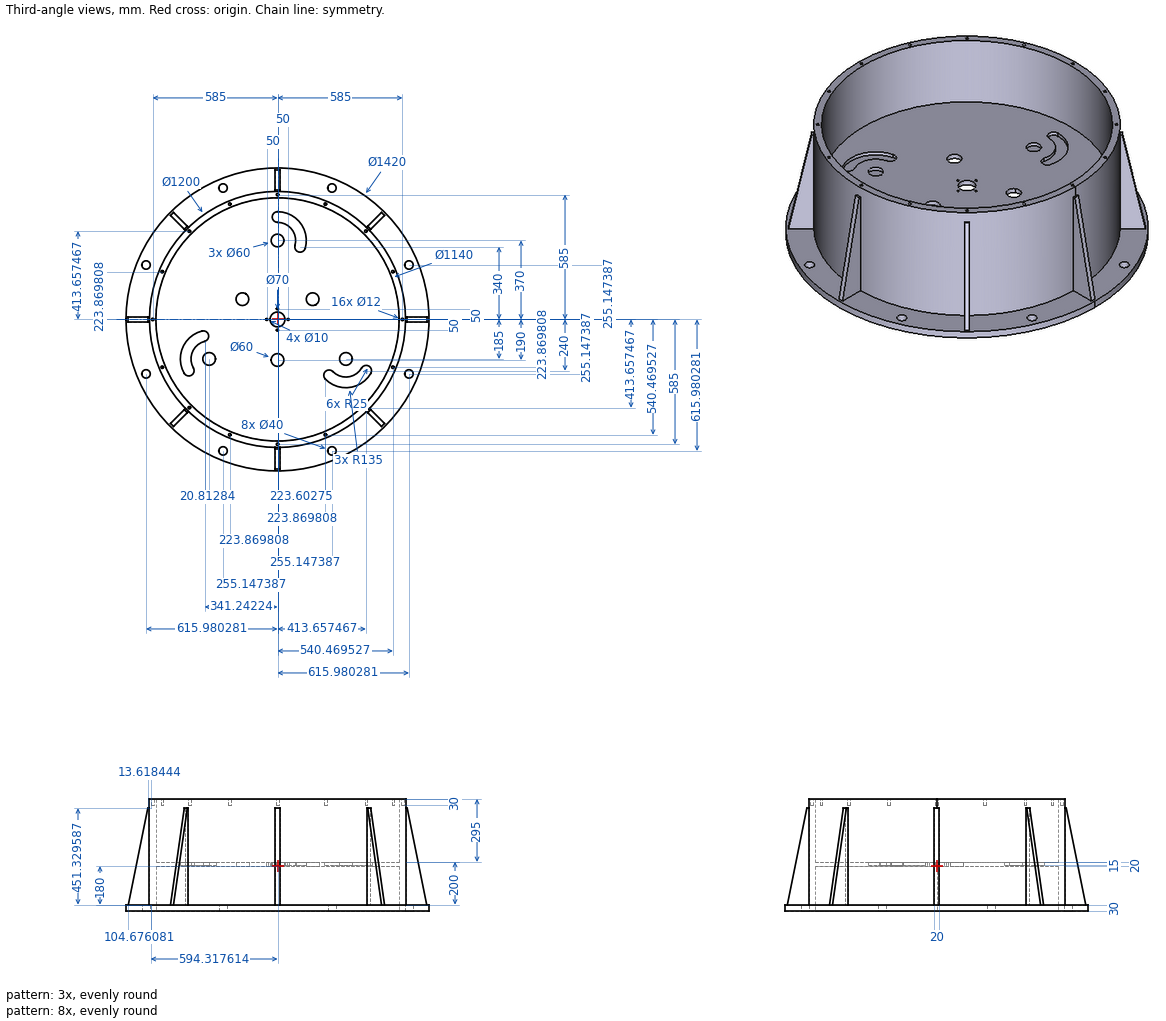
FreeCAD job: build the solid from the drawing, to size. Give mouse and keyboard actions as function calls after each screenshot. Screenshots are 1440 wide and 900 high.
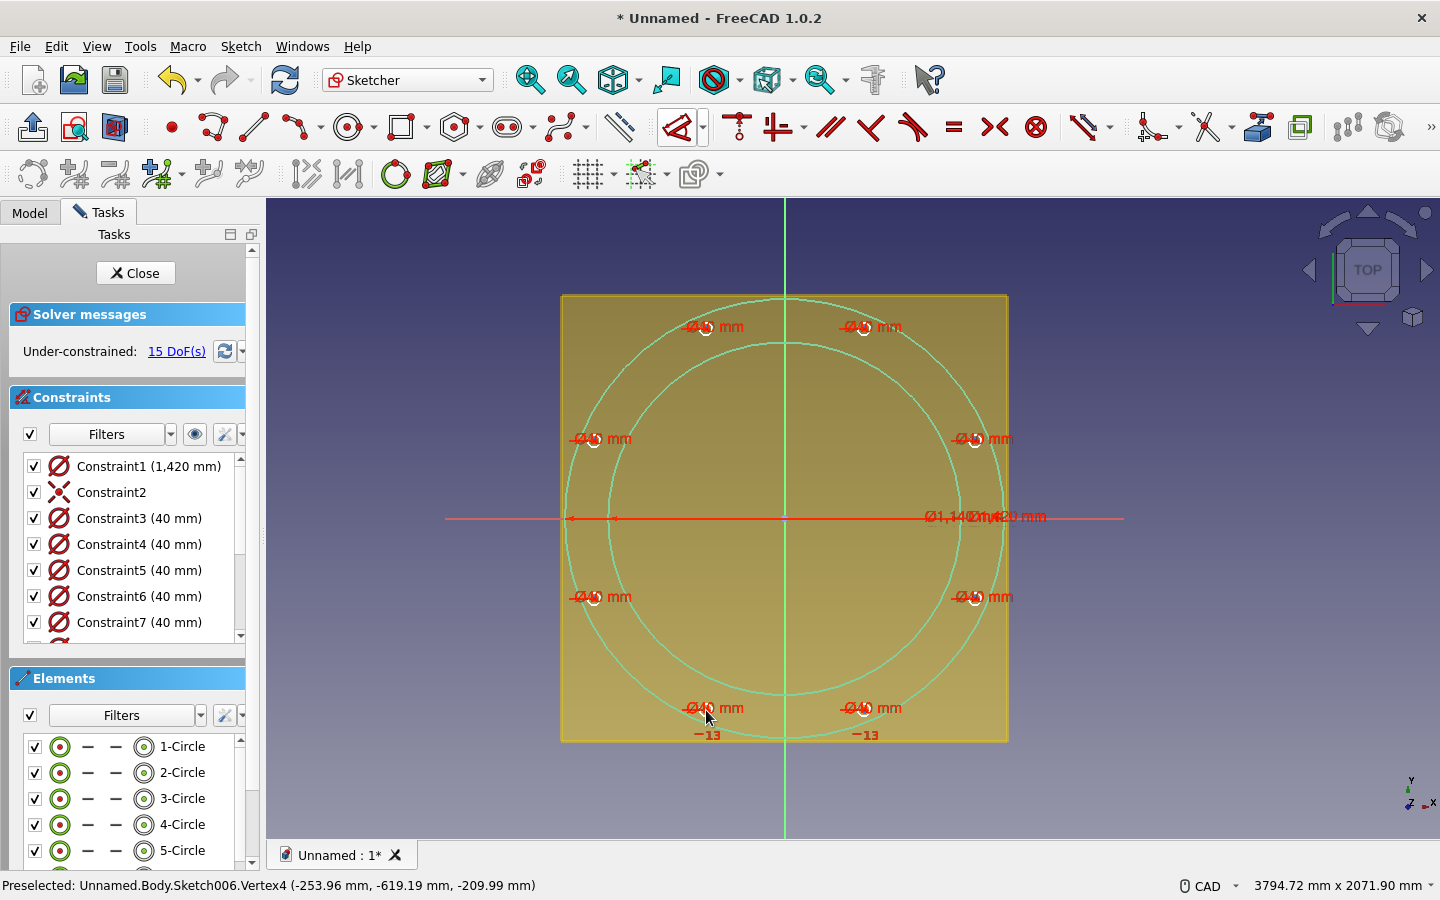
click(975, 599)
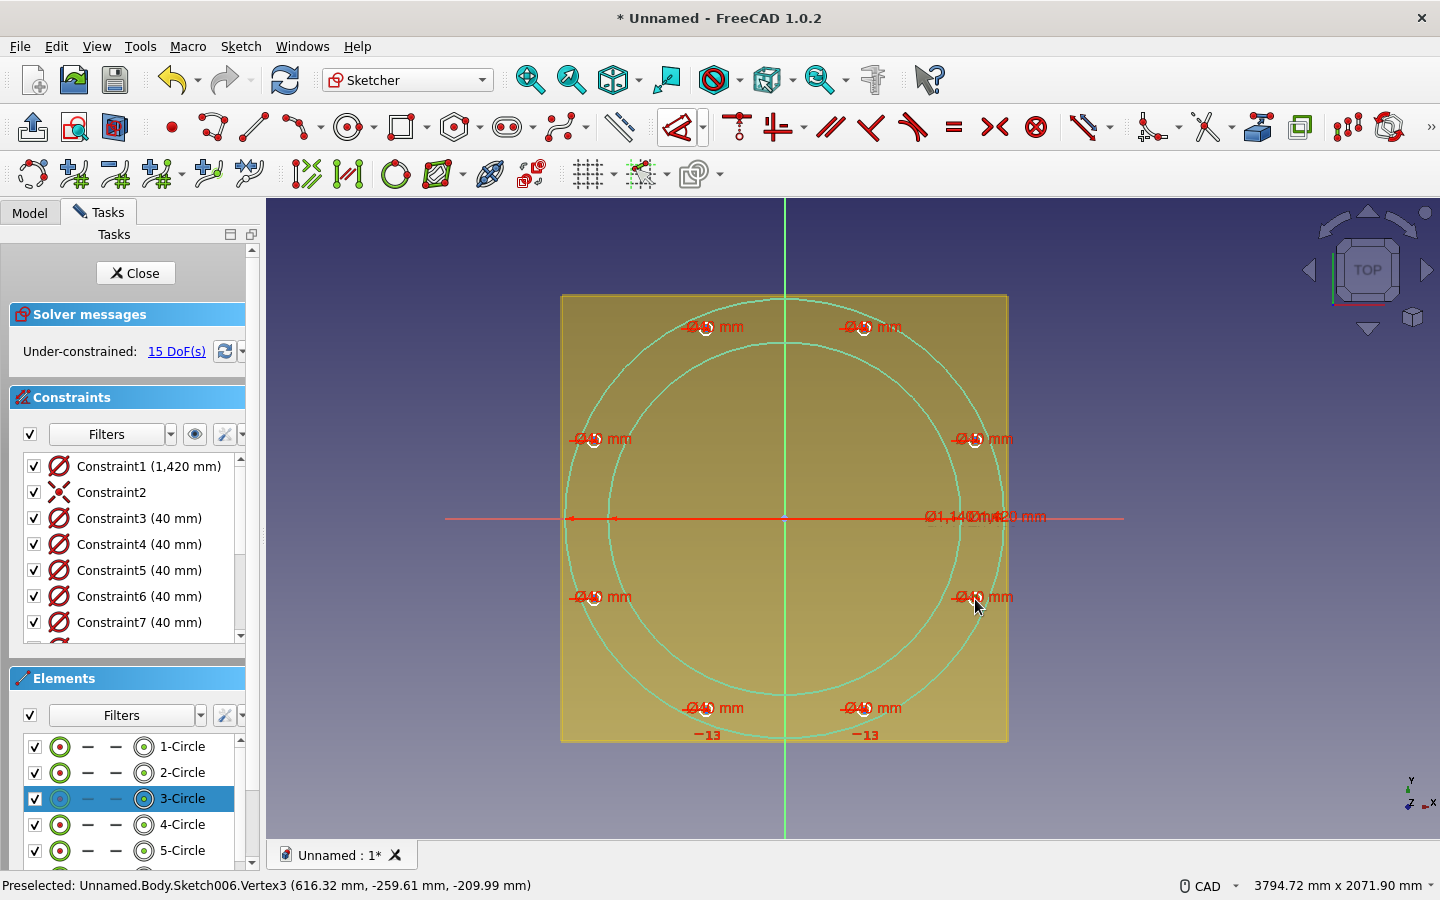
click(594, 599)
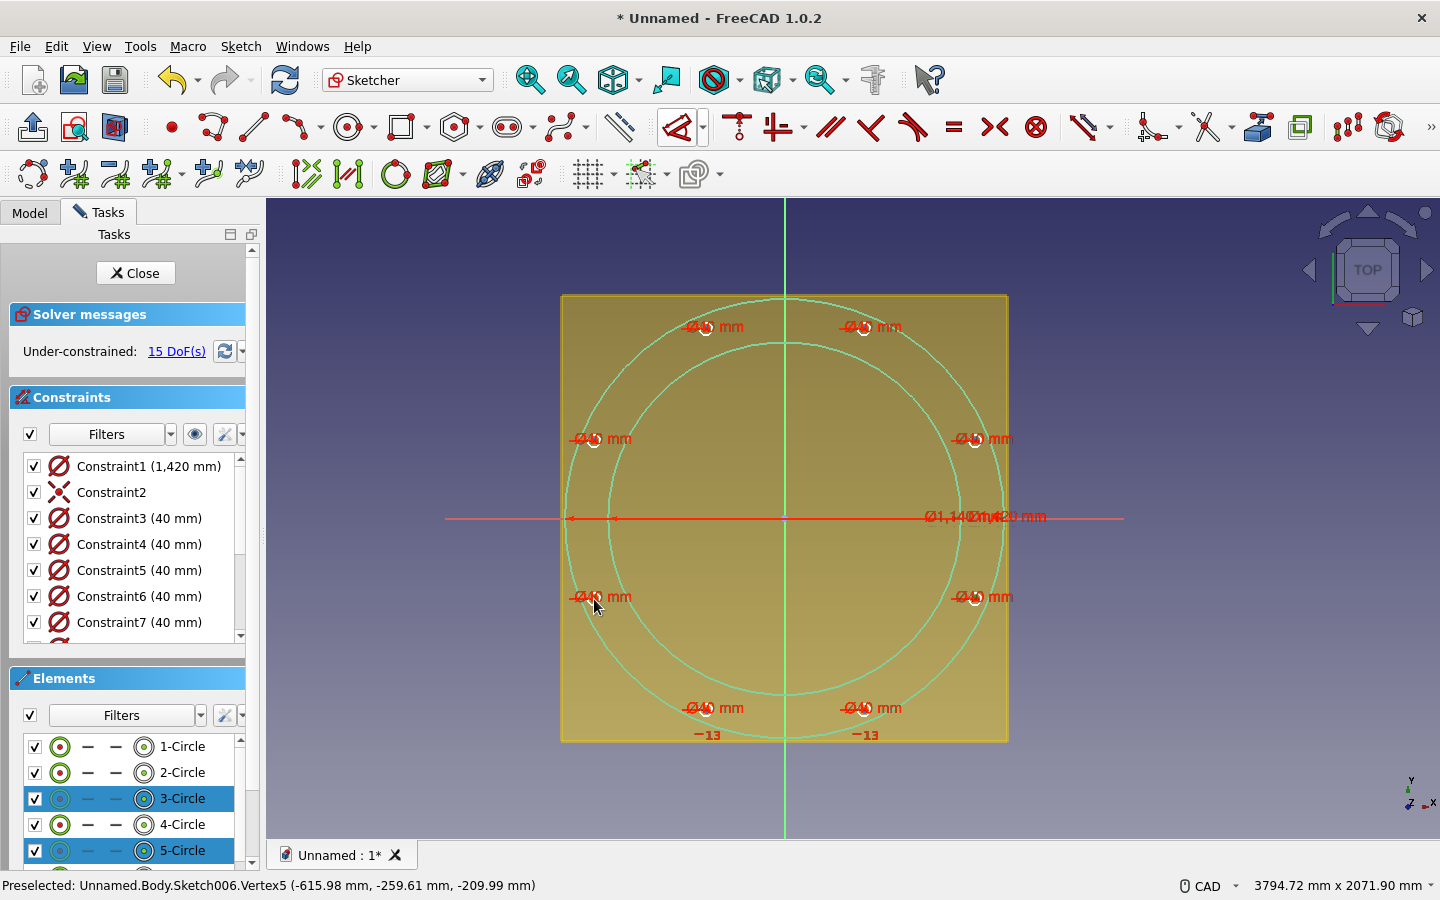
key(h)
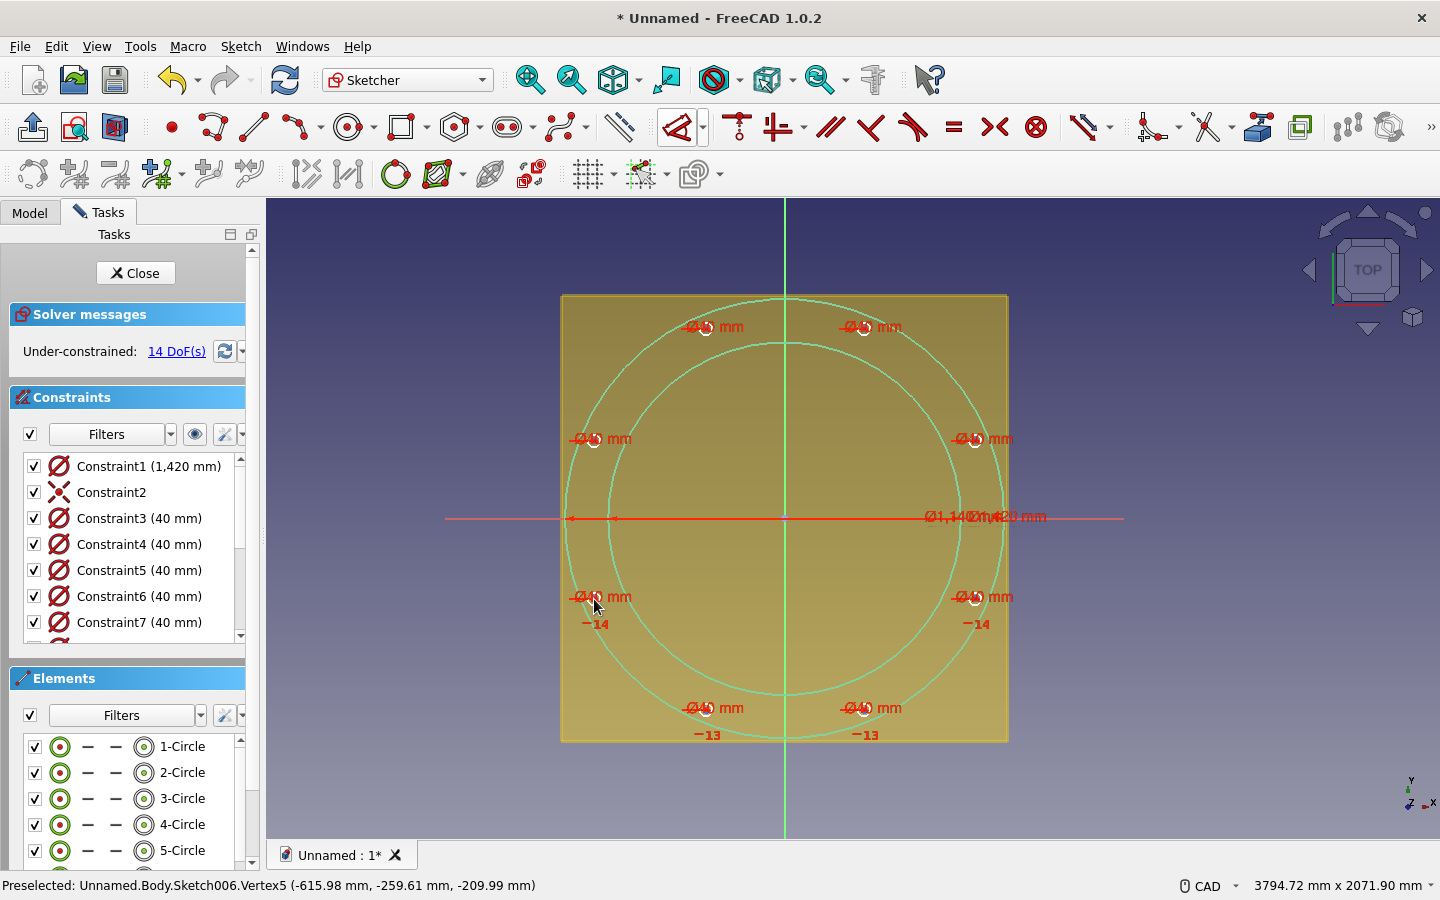
click(975, 599)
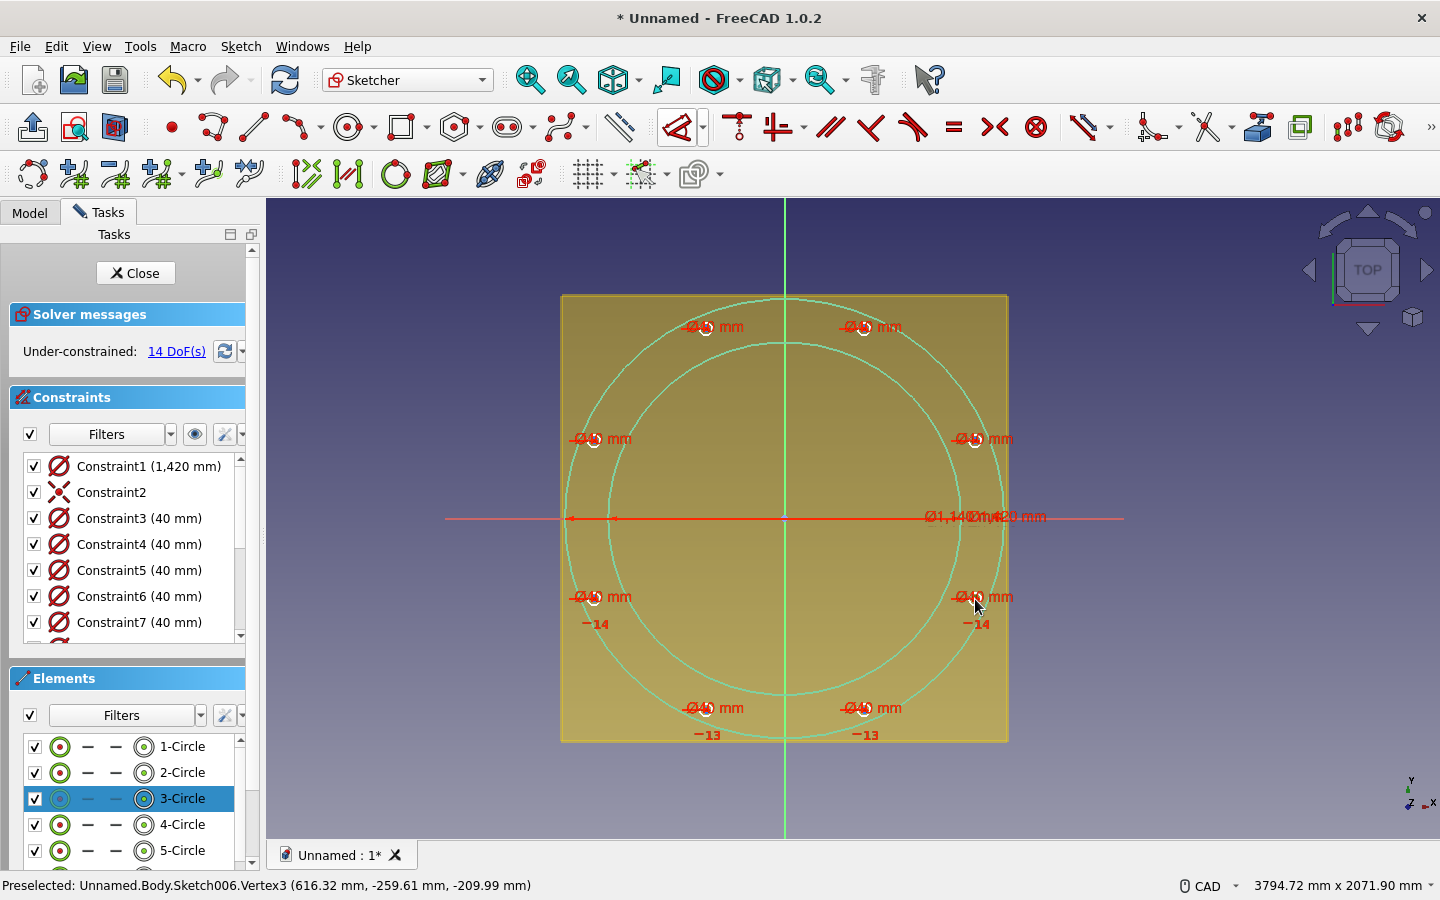
click(975, 441)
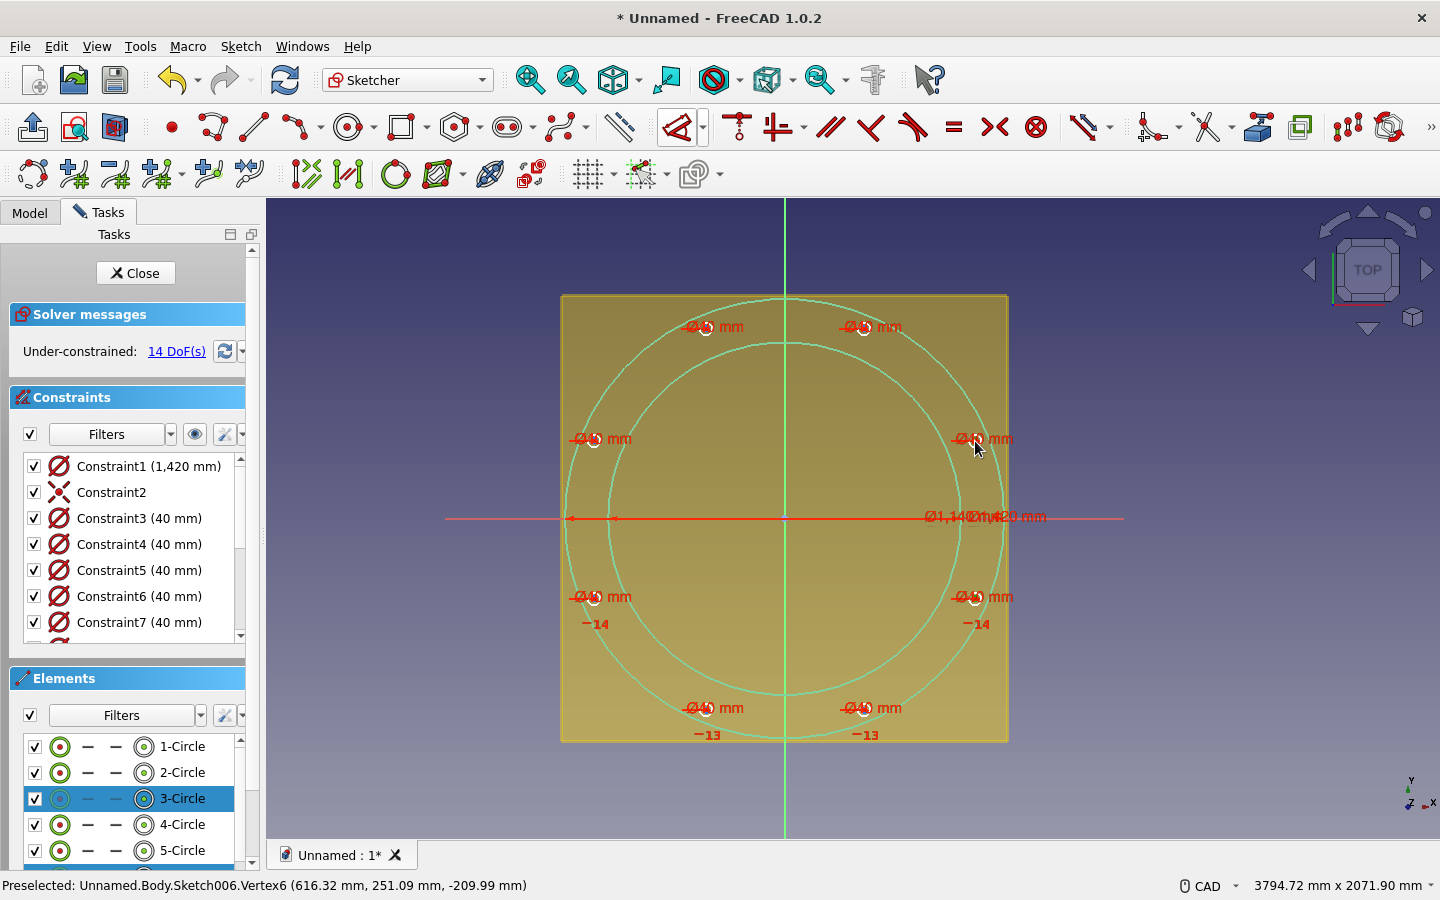
key(v)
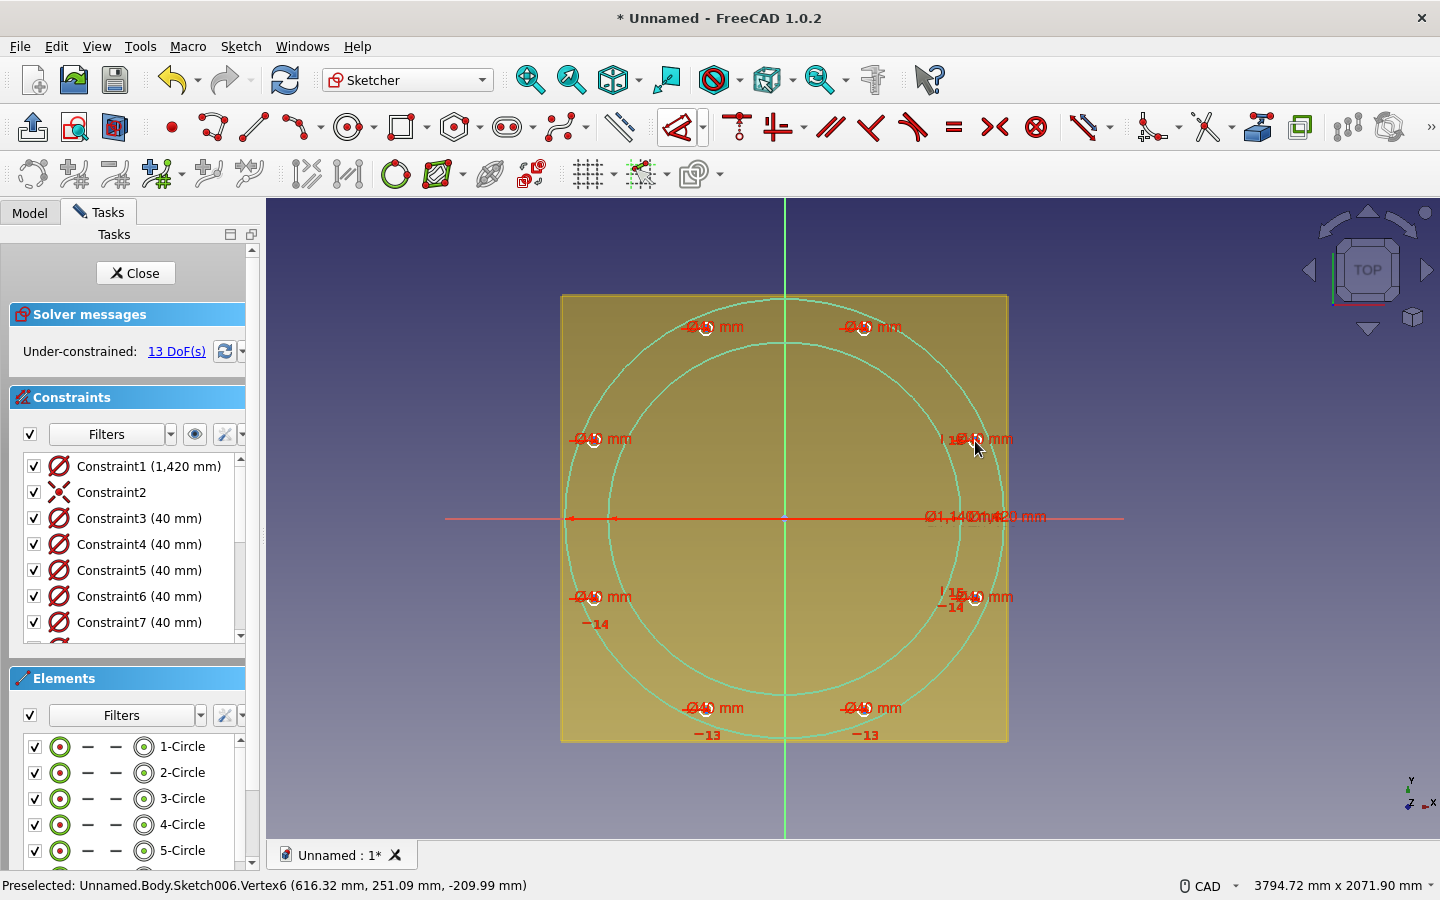
click(864, 710)